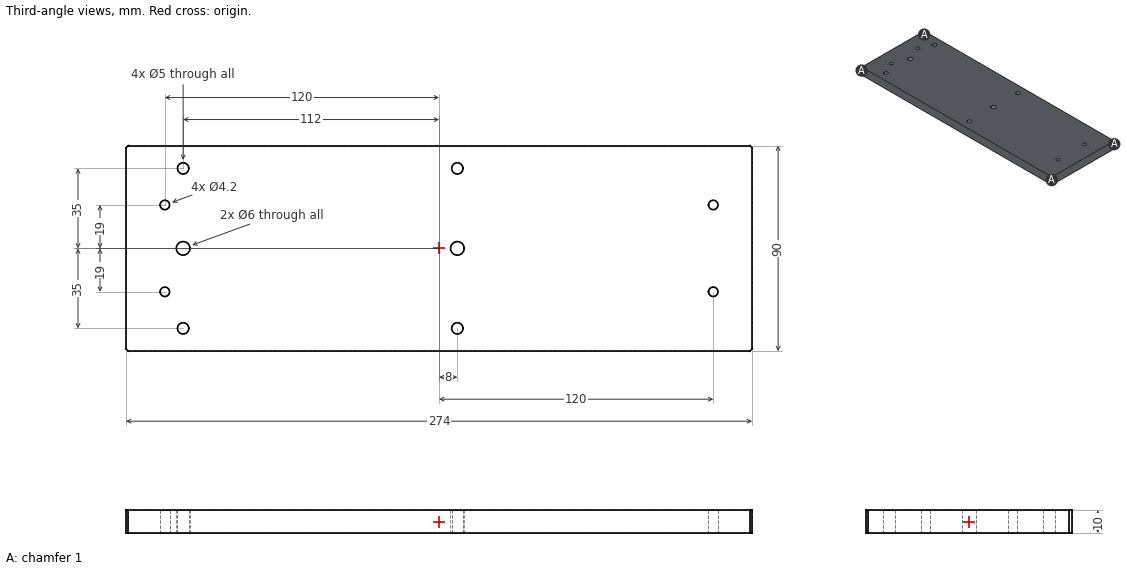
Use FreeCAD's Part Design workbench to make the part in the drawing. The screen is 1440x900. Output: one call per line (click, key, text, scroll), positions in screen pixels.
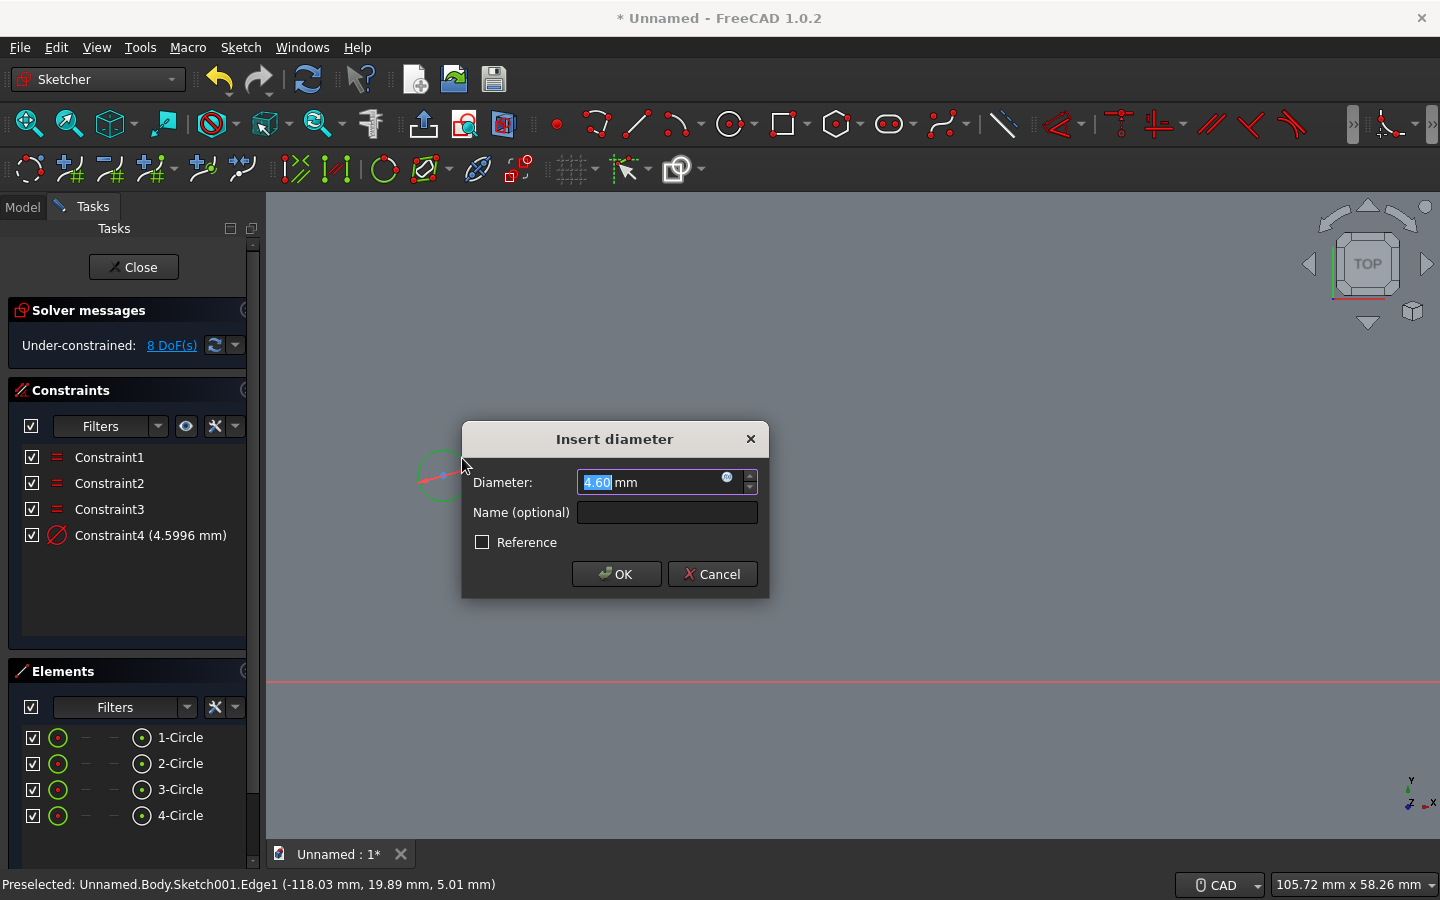
text(4.2)
key(Return)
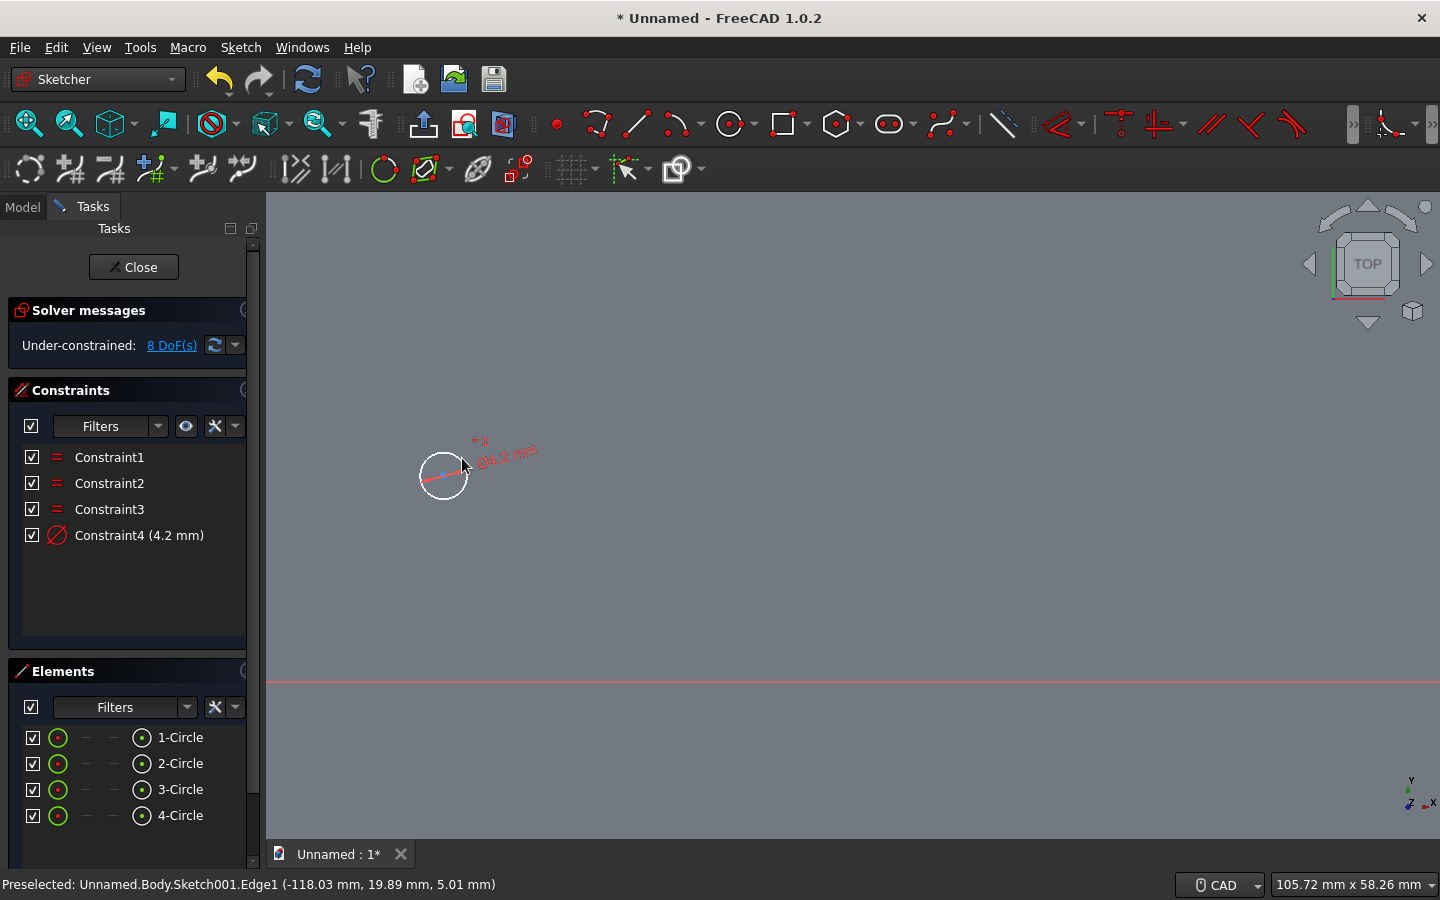
scroll(460, 461, down, 7)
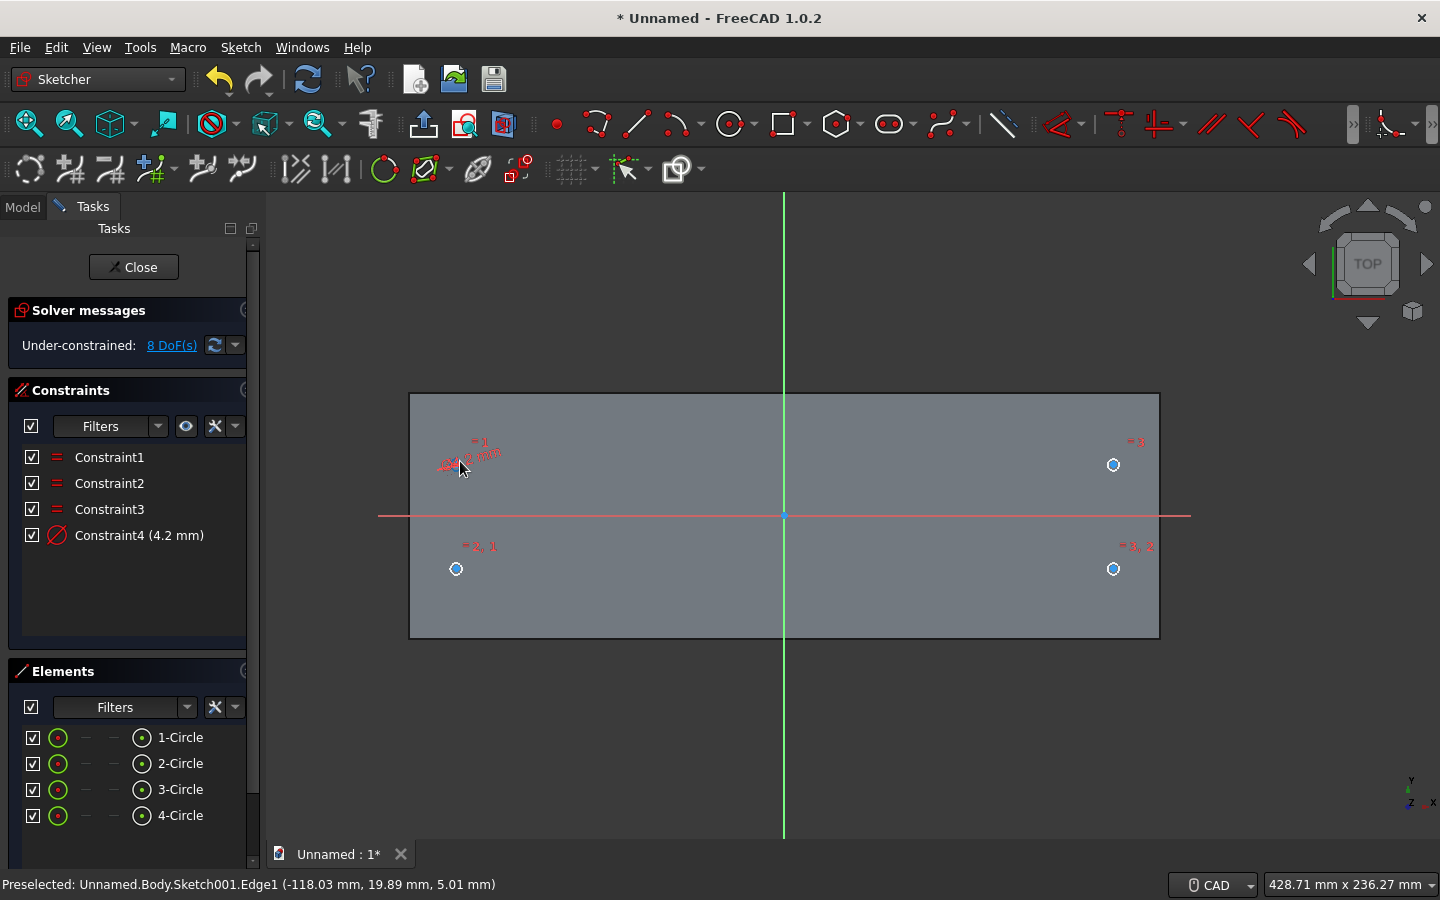
click(456, 465)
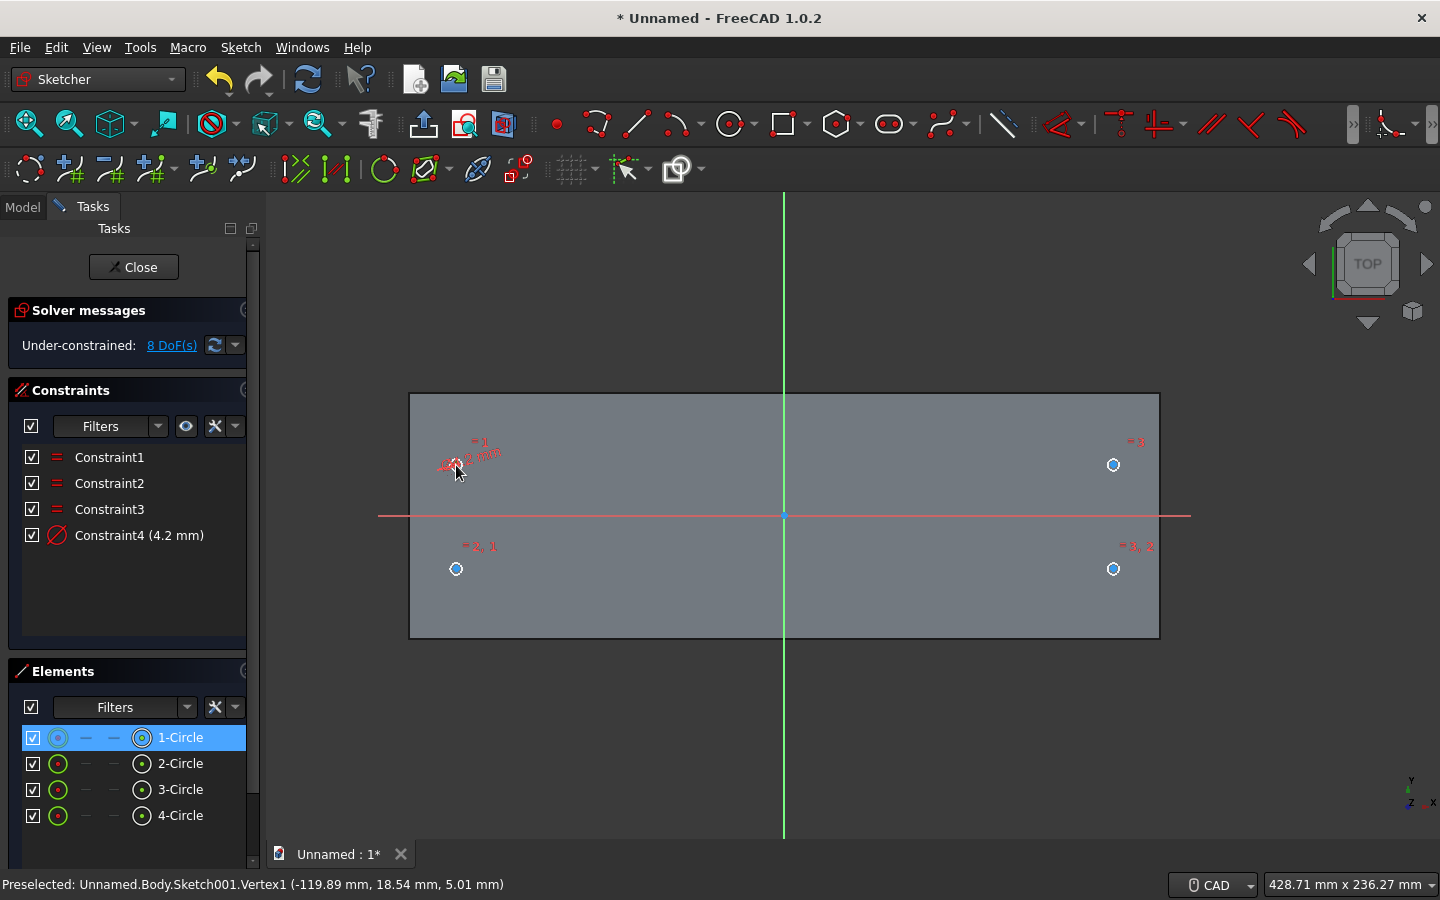
click(1084, 124)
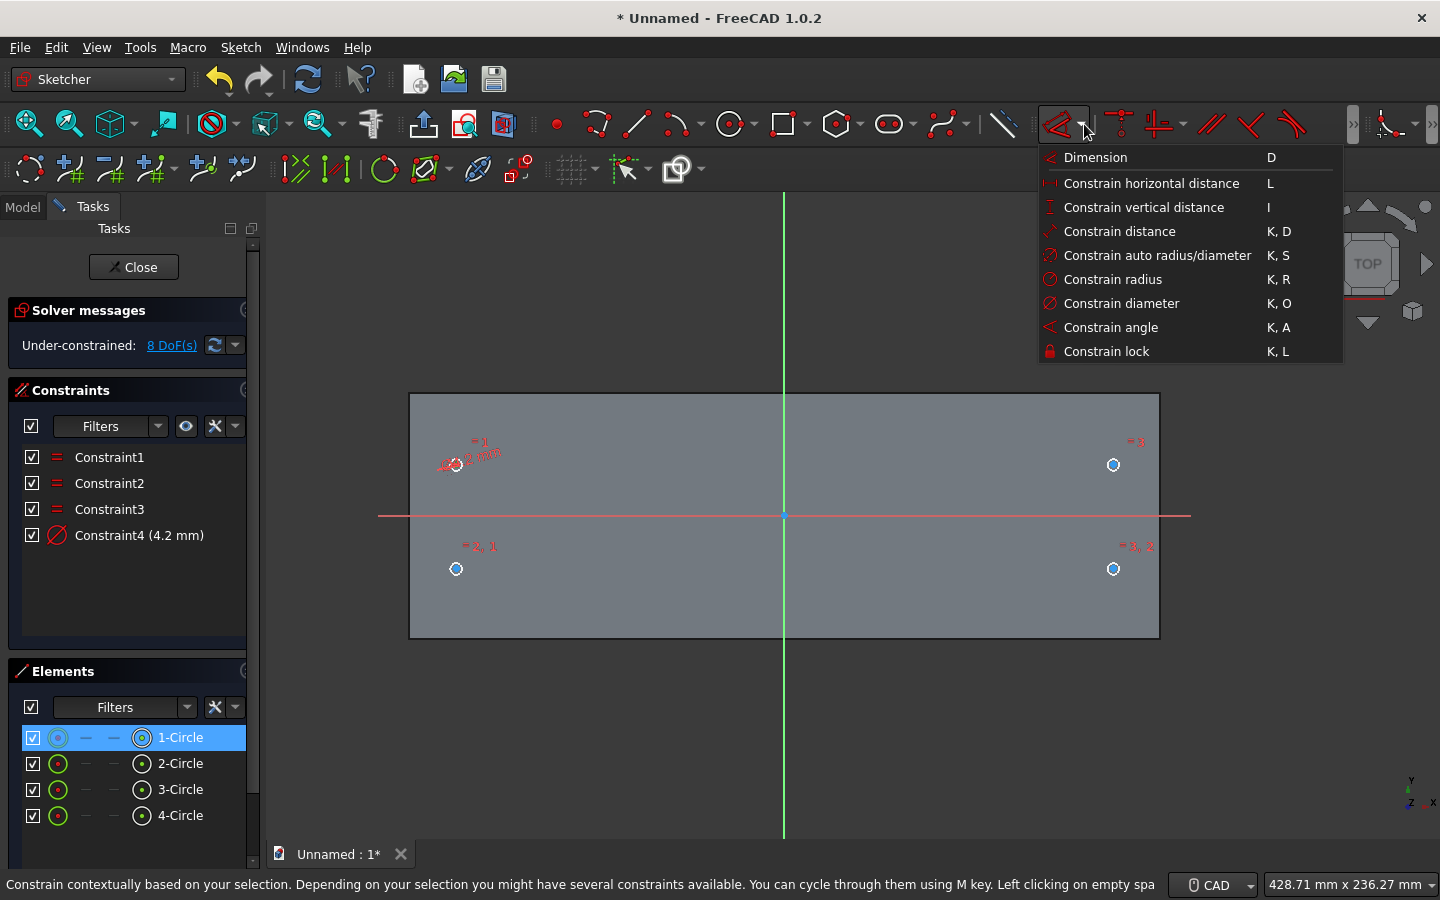
click(1191, 207)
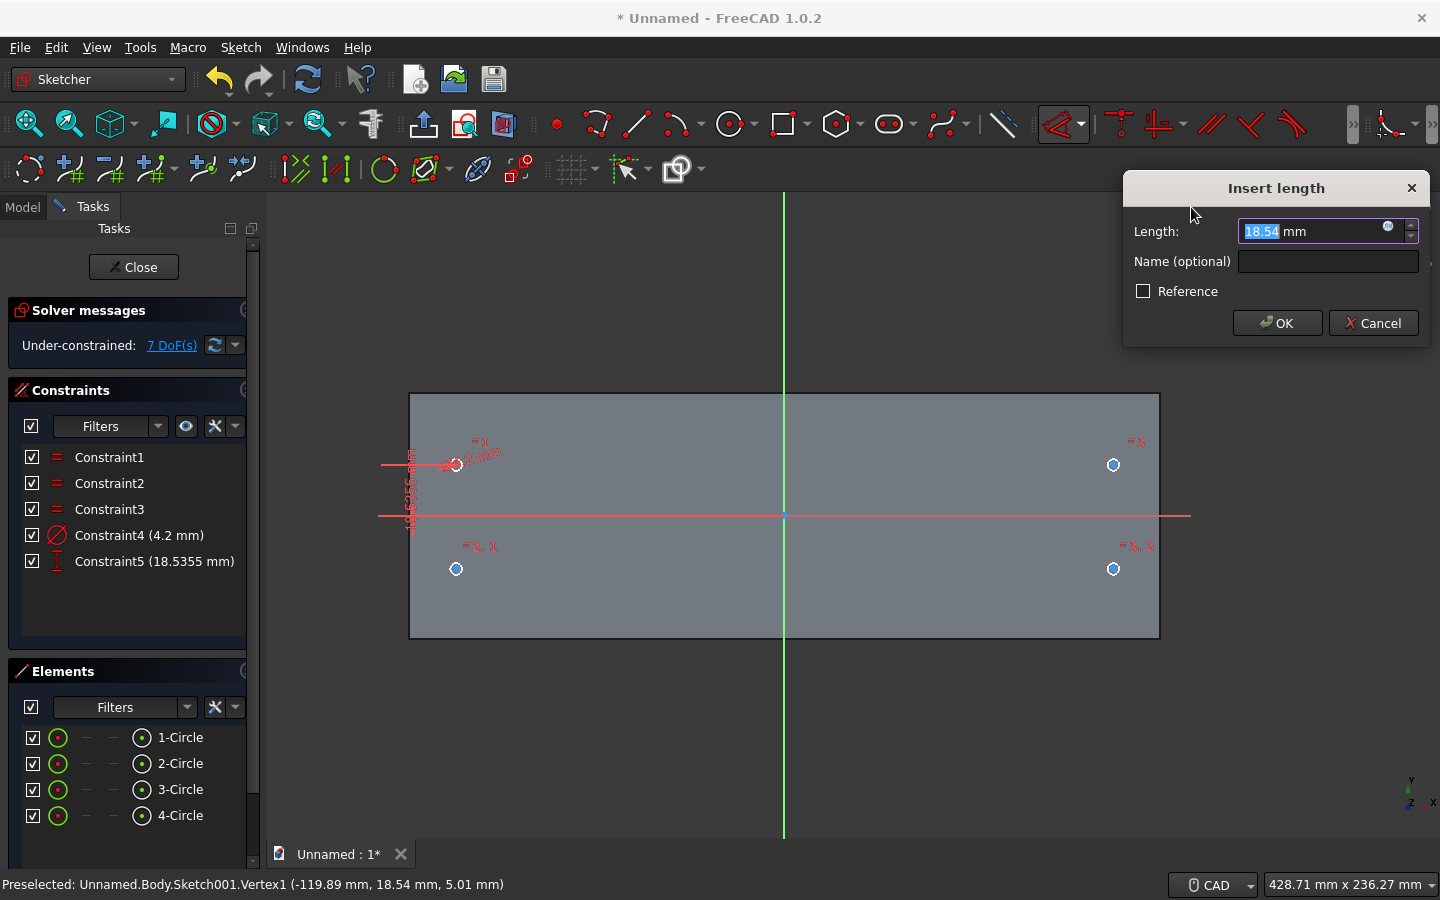
text(19)
key(Return)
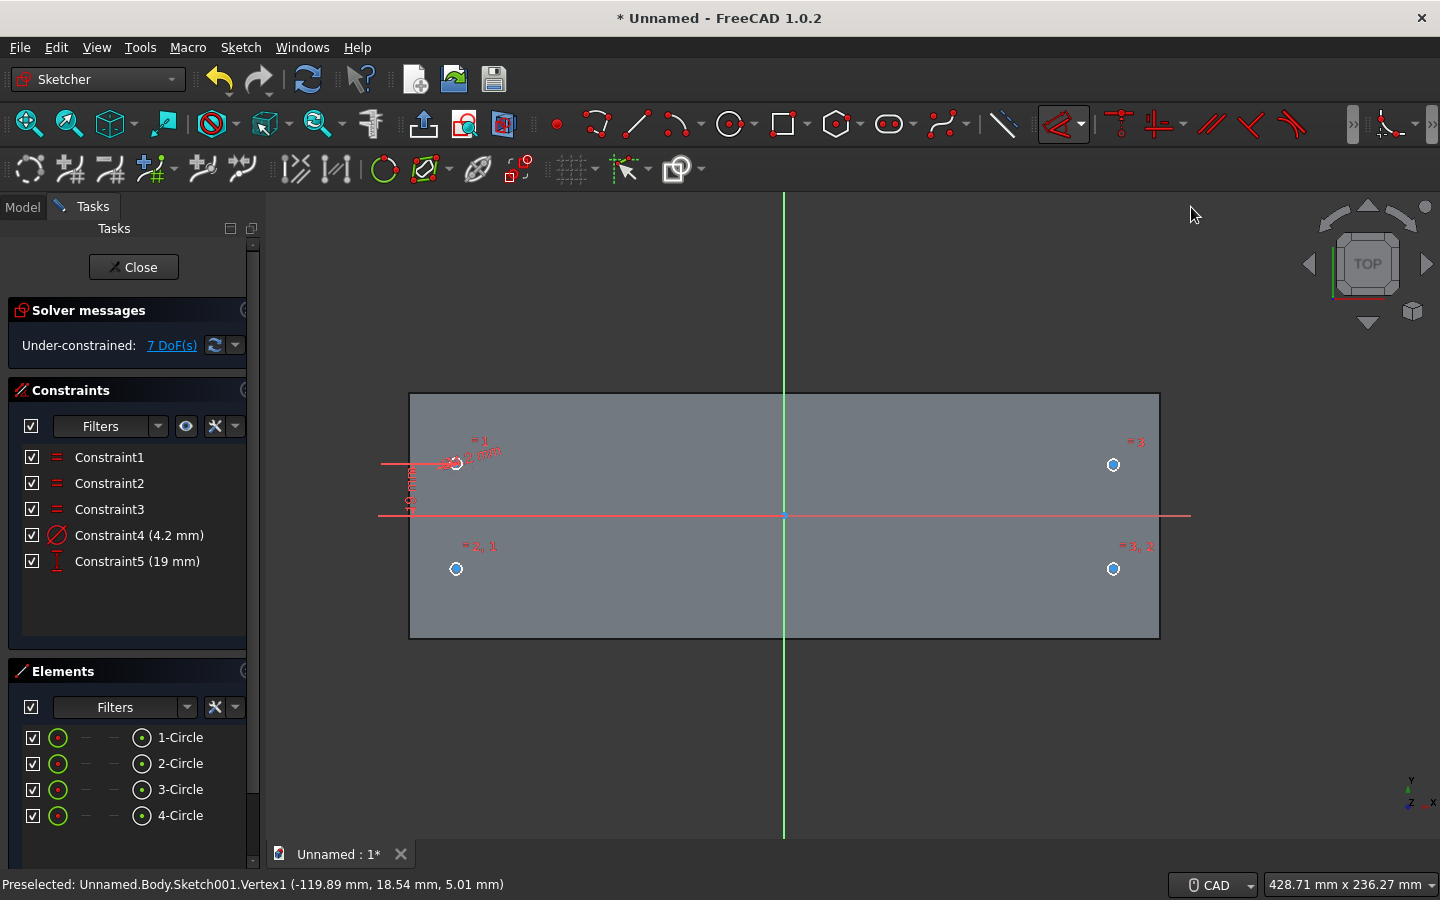
click(456, 569)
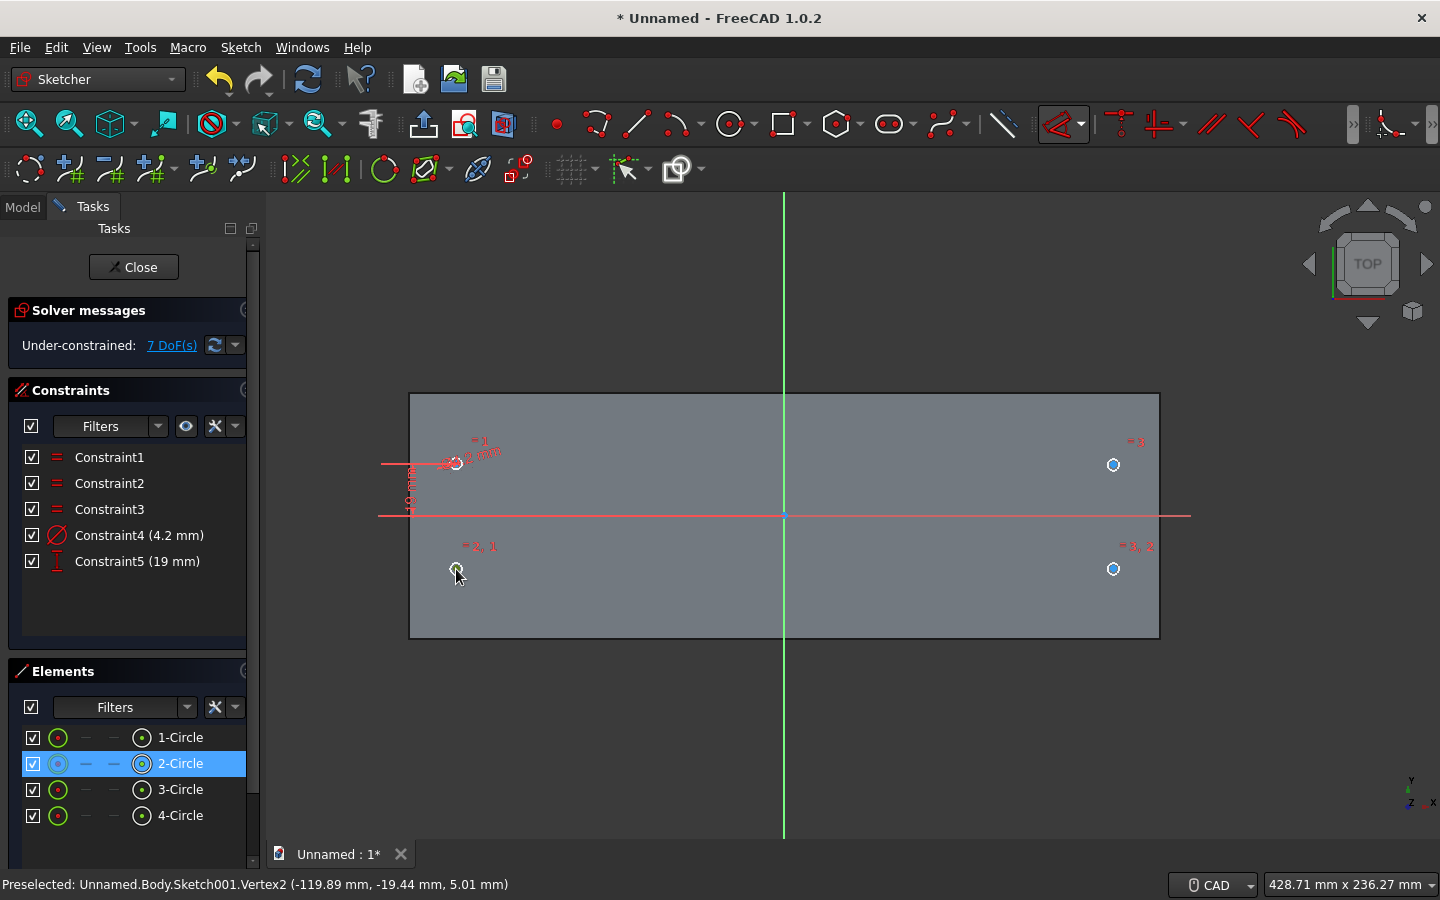
key(i)